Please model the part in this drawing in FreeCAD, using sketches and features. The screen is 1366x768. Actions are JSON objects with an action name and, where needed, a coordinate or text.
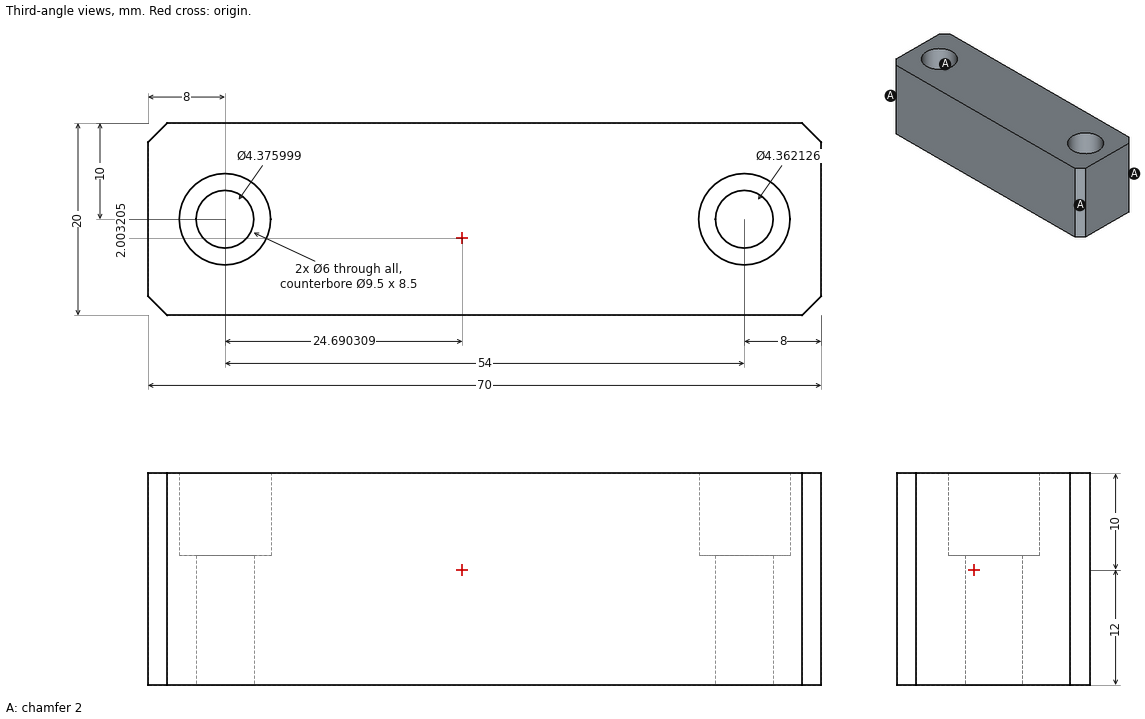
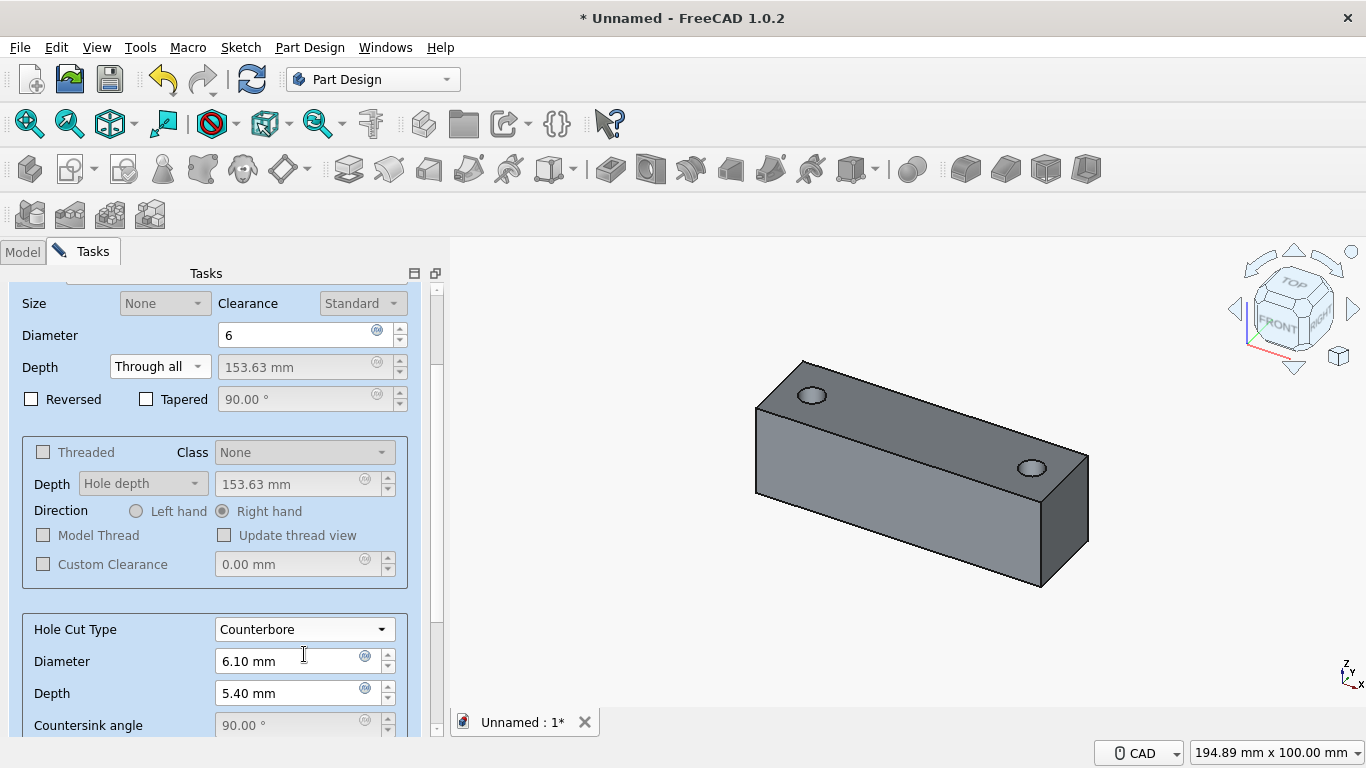
{"action": "triple_click", "coordinate": [298, 661]}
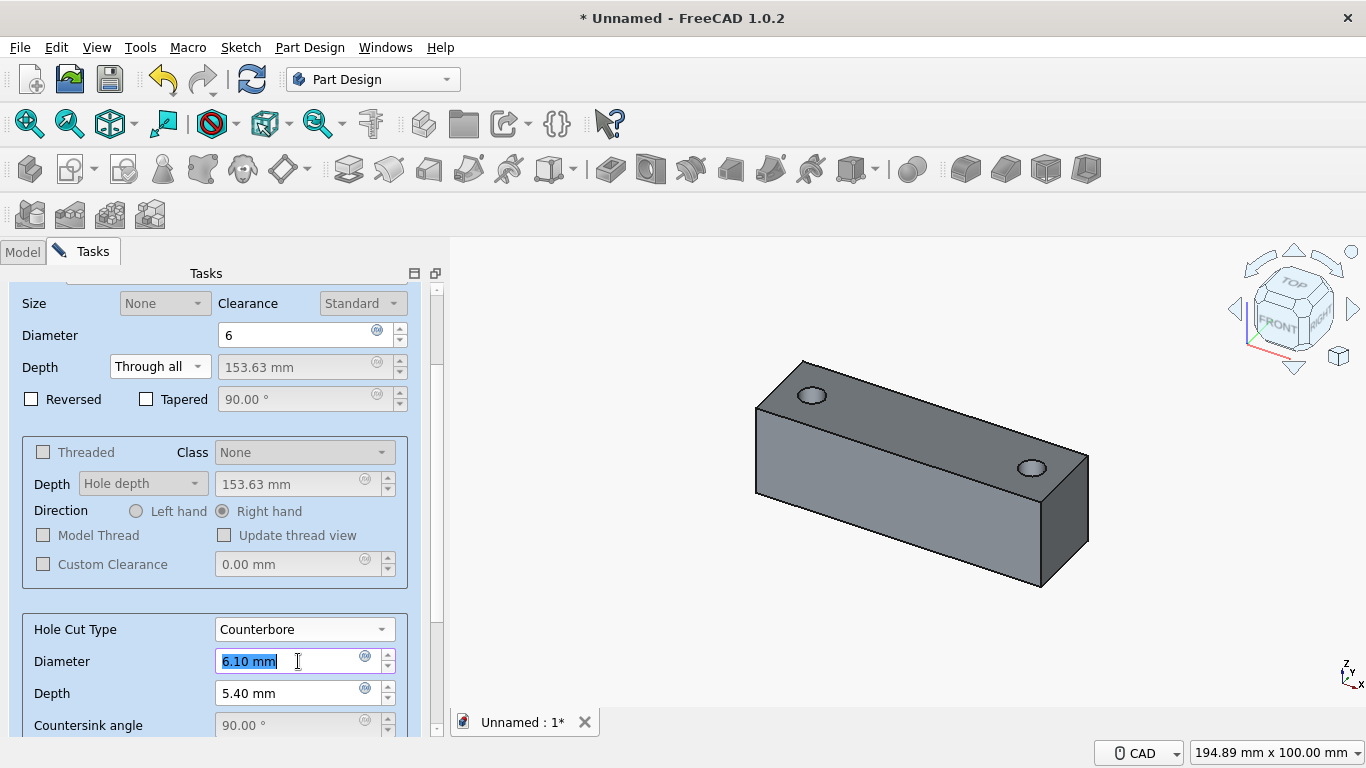
{"action": "type", "text": "9.5"}
{"action": "key", "text": "Tab"}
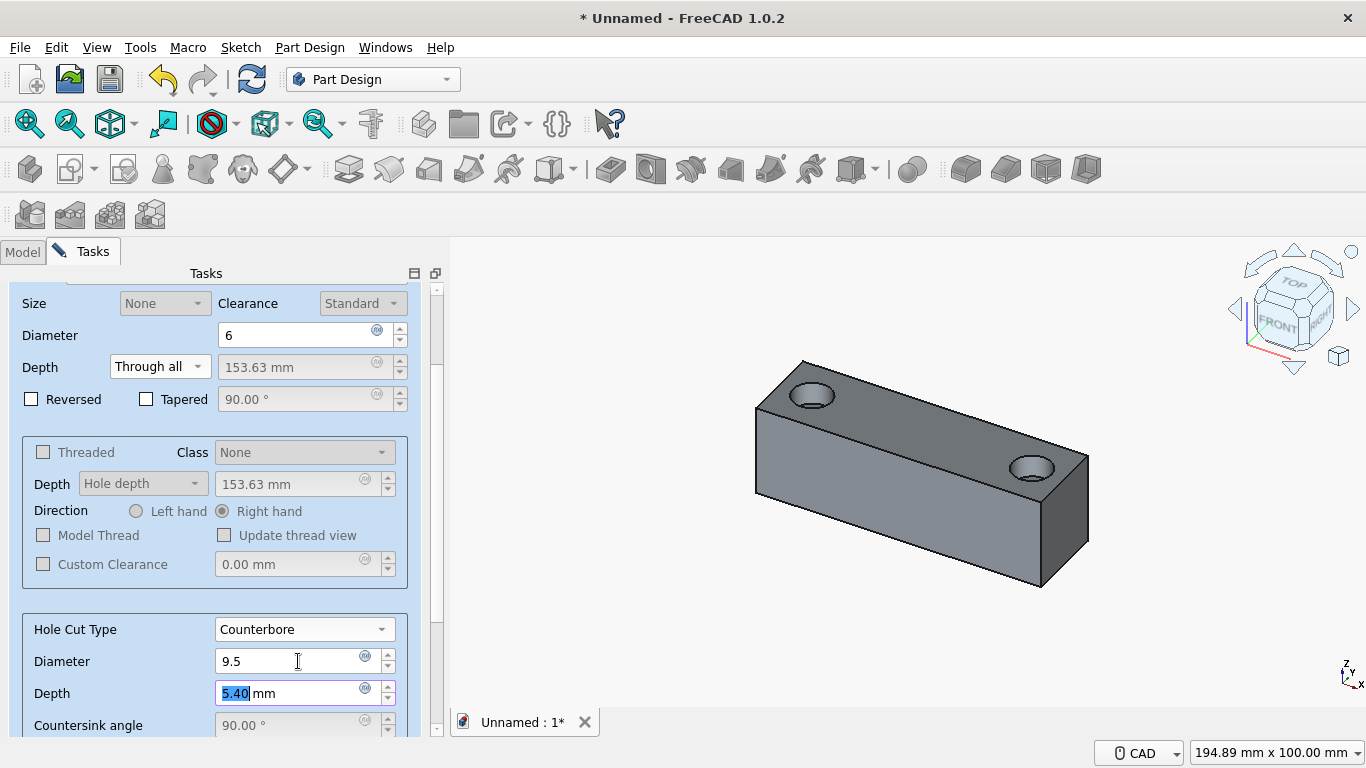
{"action": "type", "text": "8.5"}
{"action": "key", "text": "Tab"}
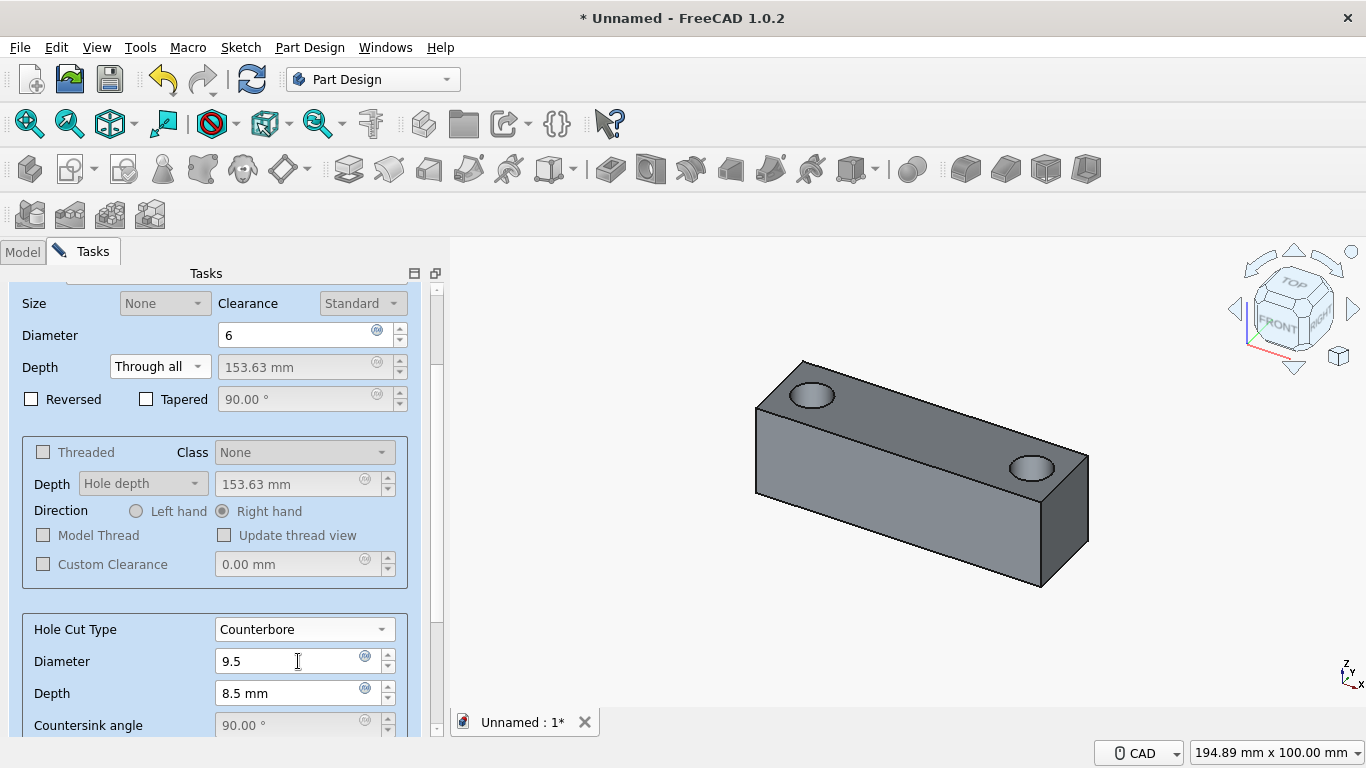
{"action": "scroll", "coordinate": [437, 510], "scroll_direction": "up", "scroll_amount": 3}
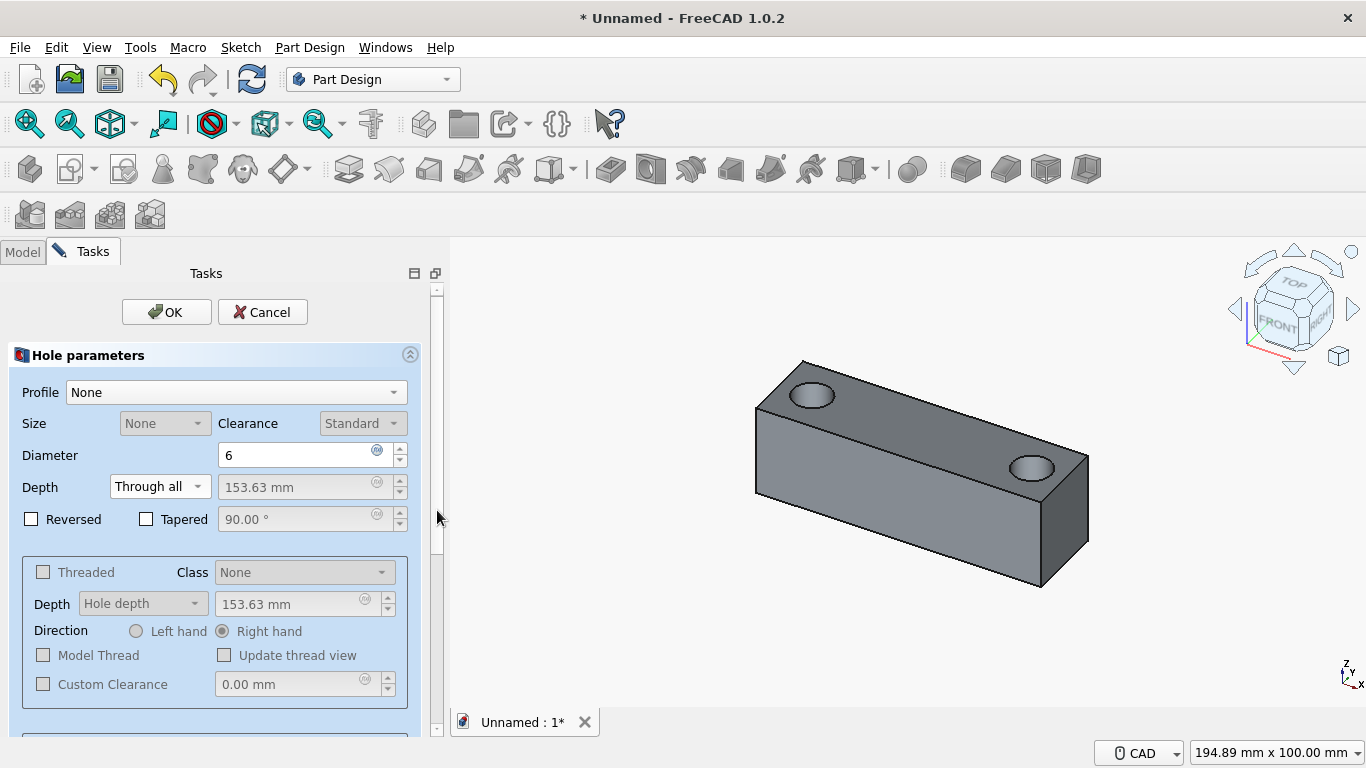
{"action": "left_click", "coordinate": [167, 312]}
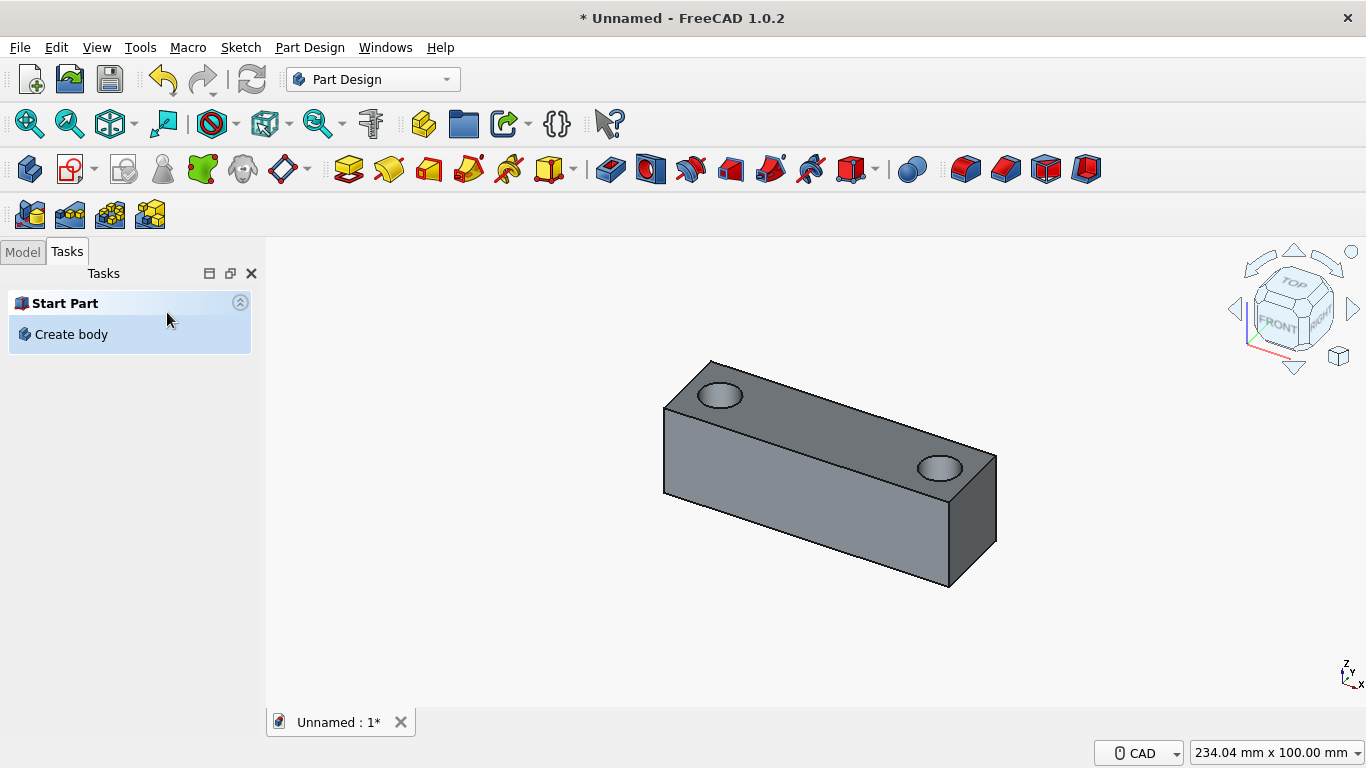
{"action": "left_click", "coordinate": [949, 544]}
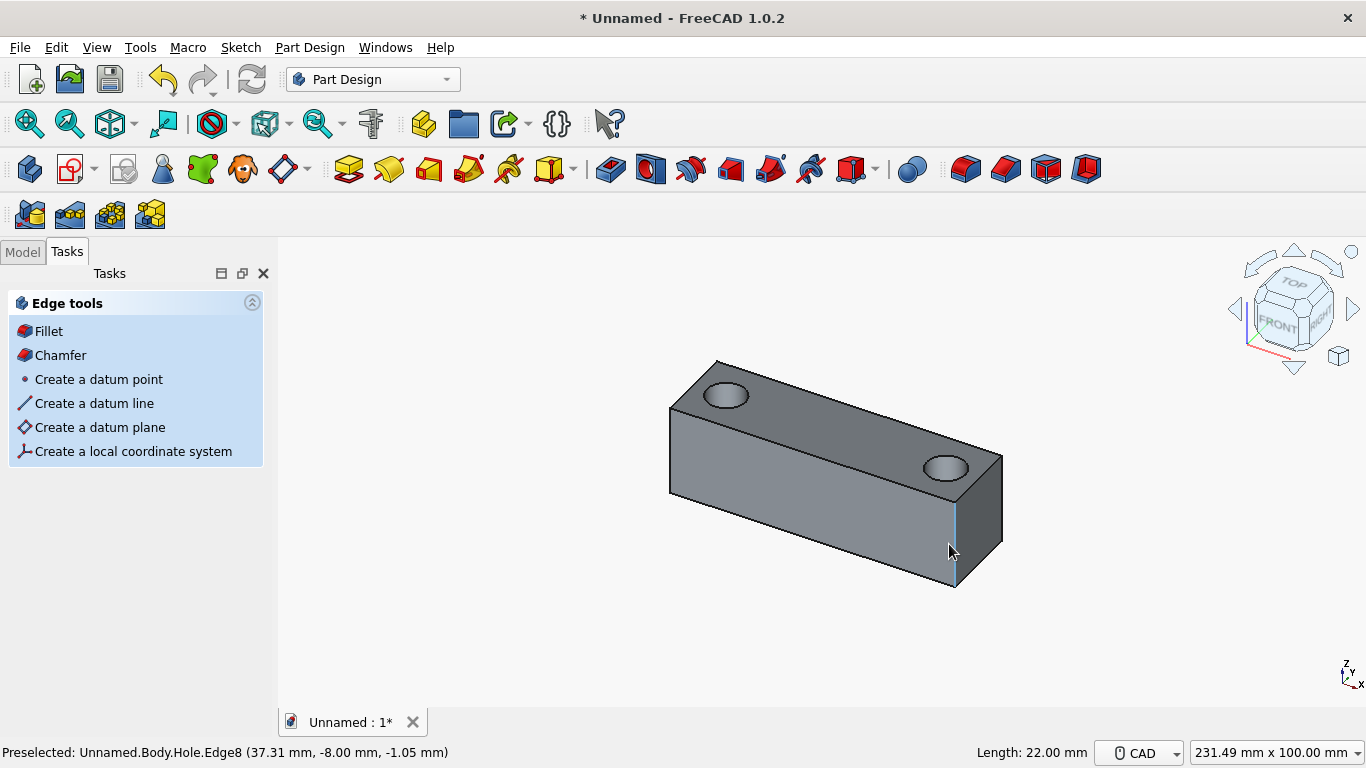
{"action": "key", "text": "0"}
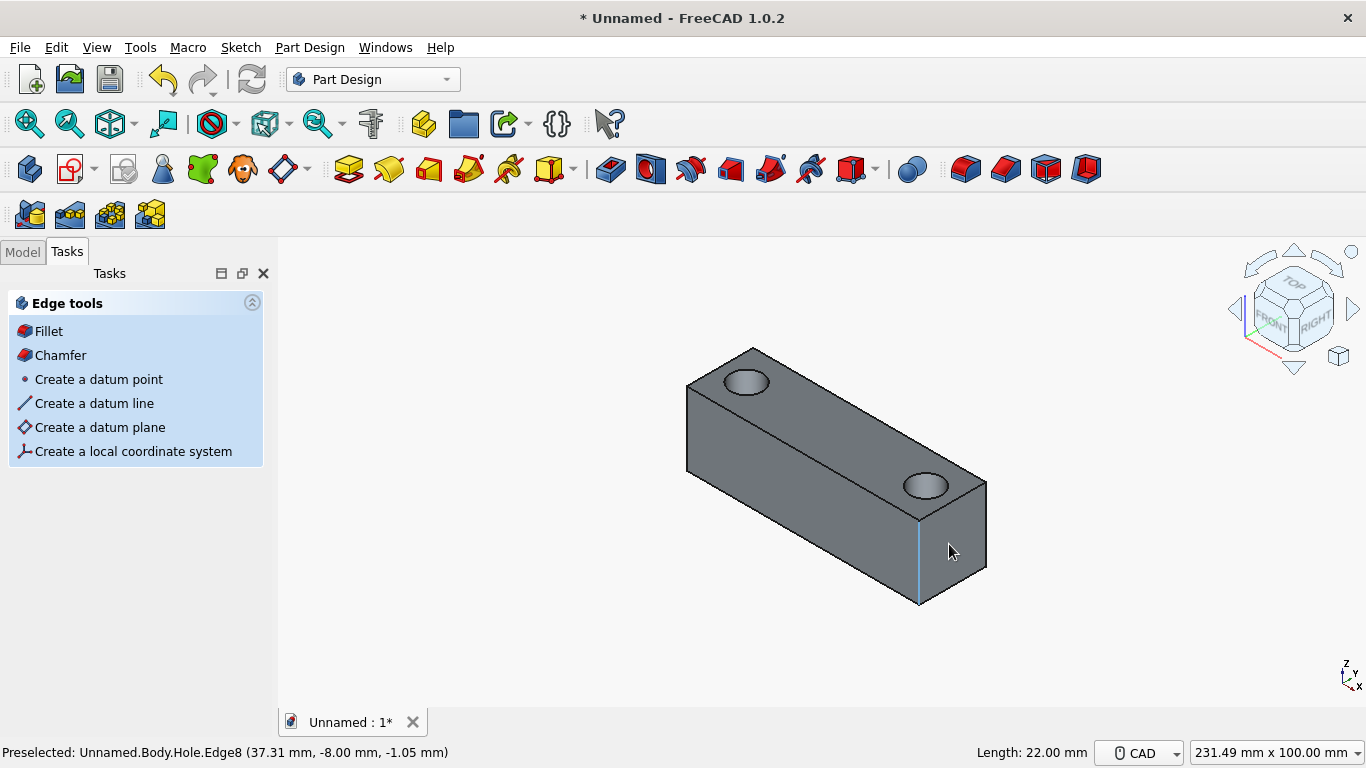
{"action": "key", "text": "2"}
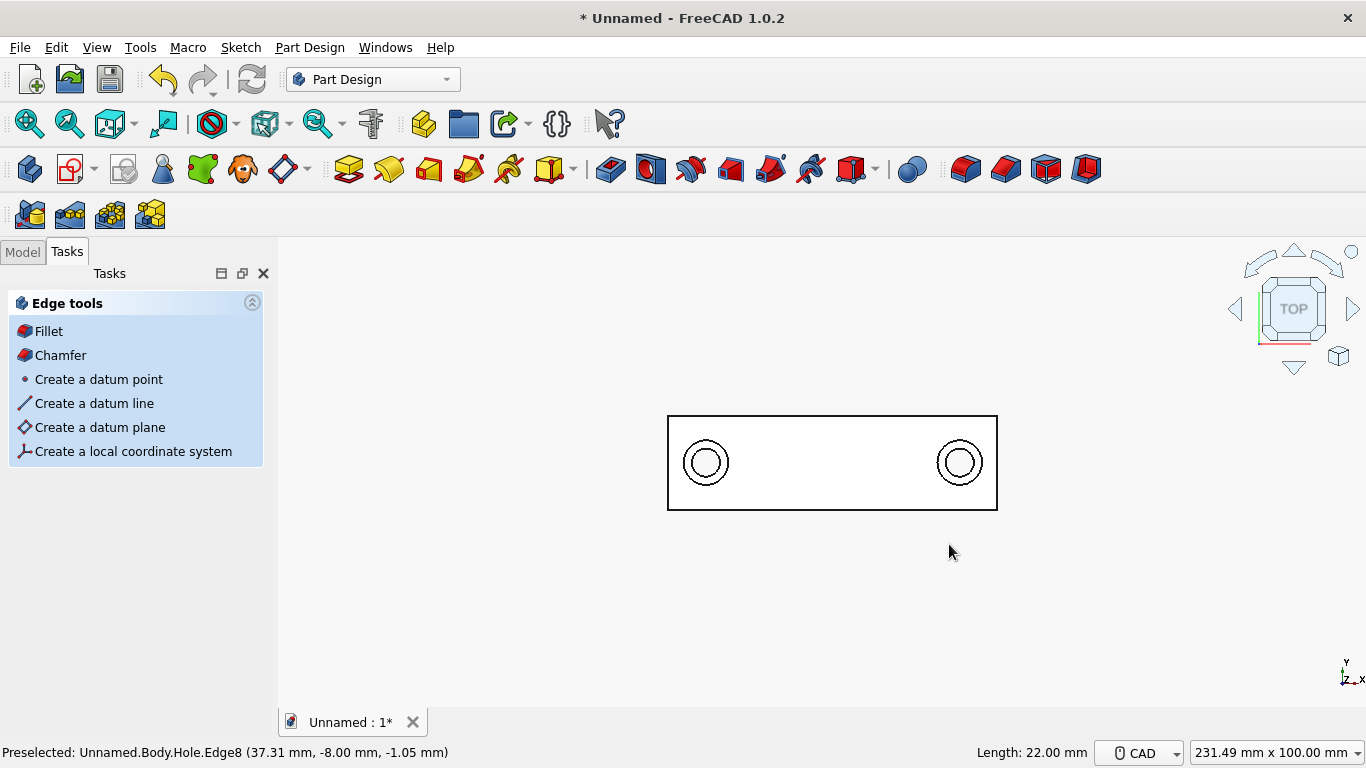
{"action": "key", "text": "v f"}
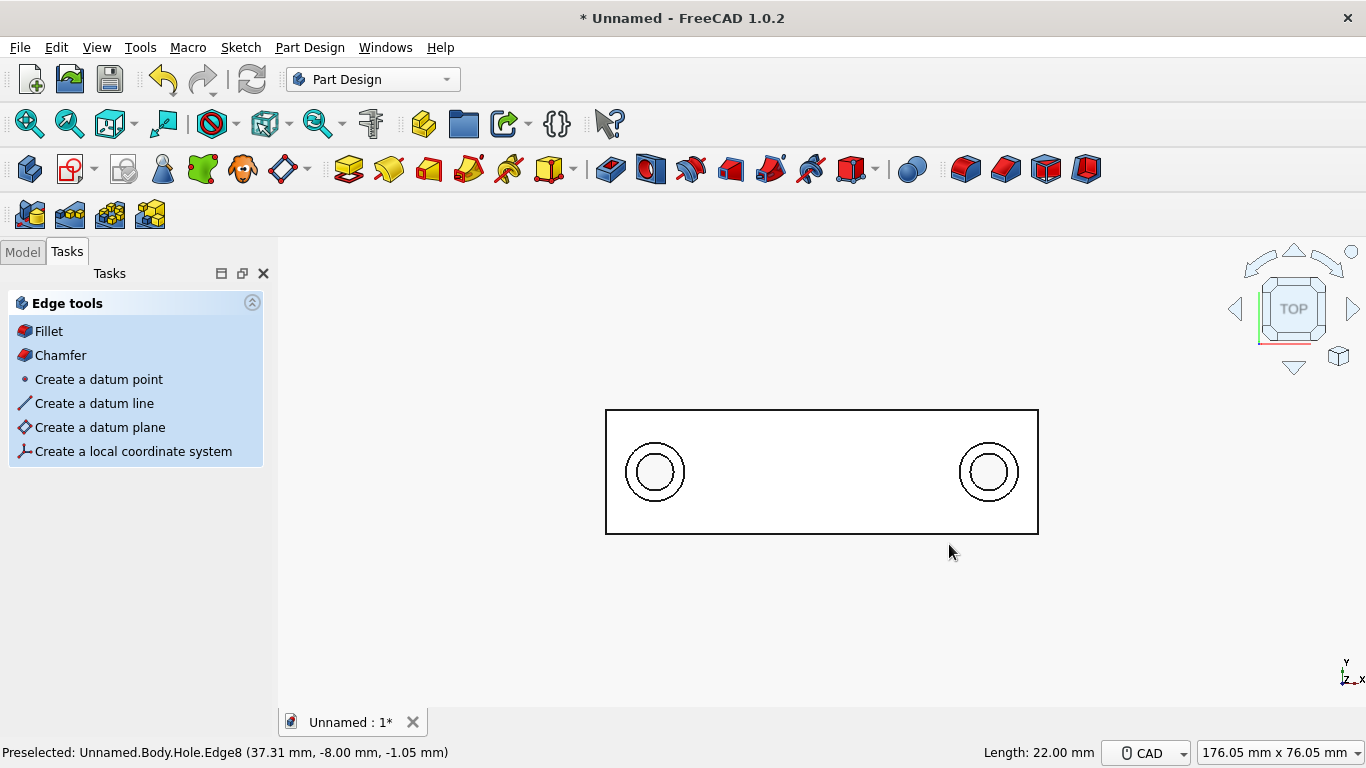
{"action": "key", "text": "1"}